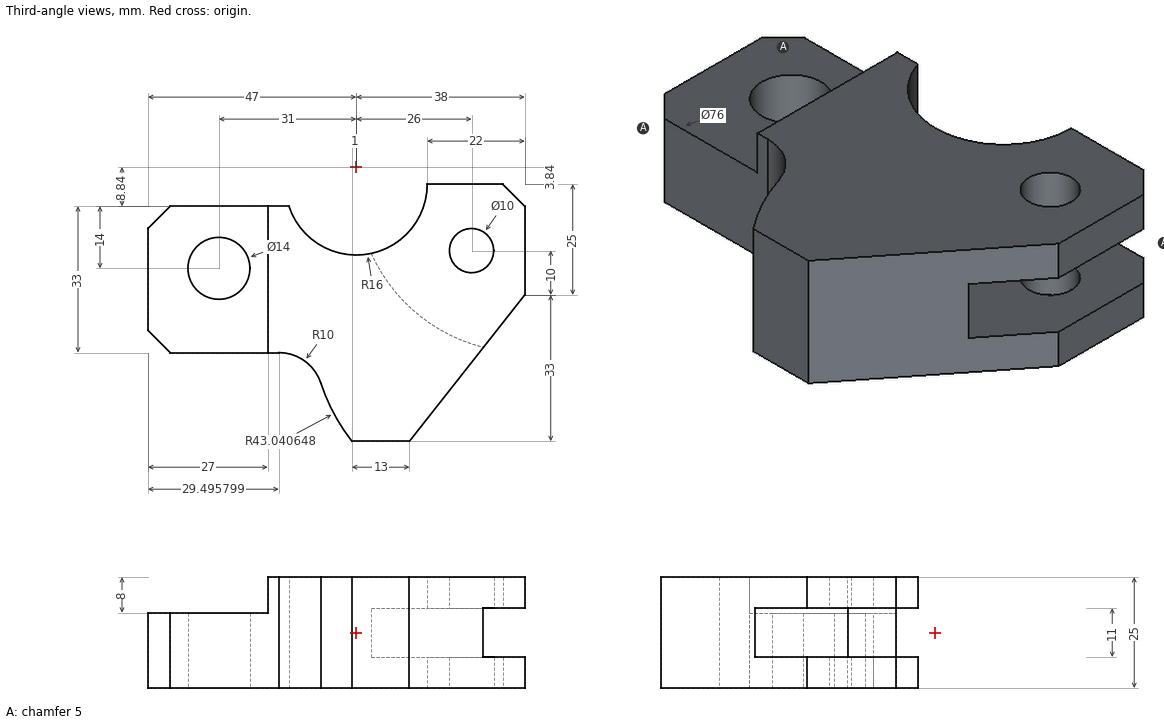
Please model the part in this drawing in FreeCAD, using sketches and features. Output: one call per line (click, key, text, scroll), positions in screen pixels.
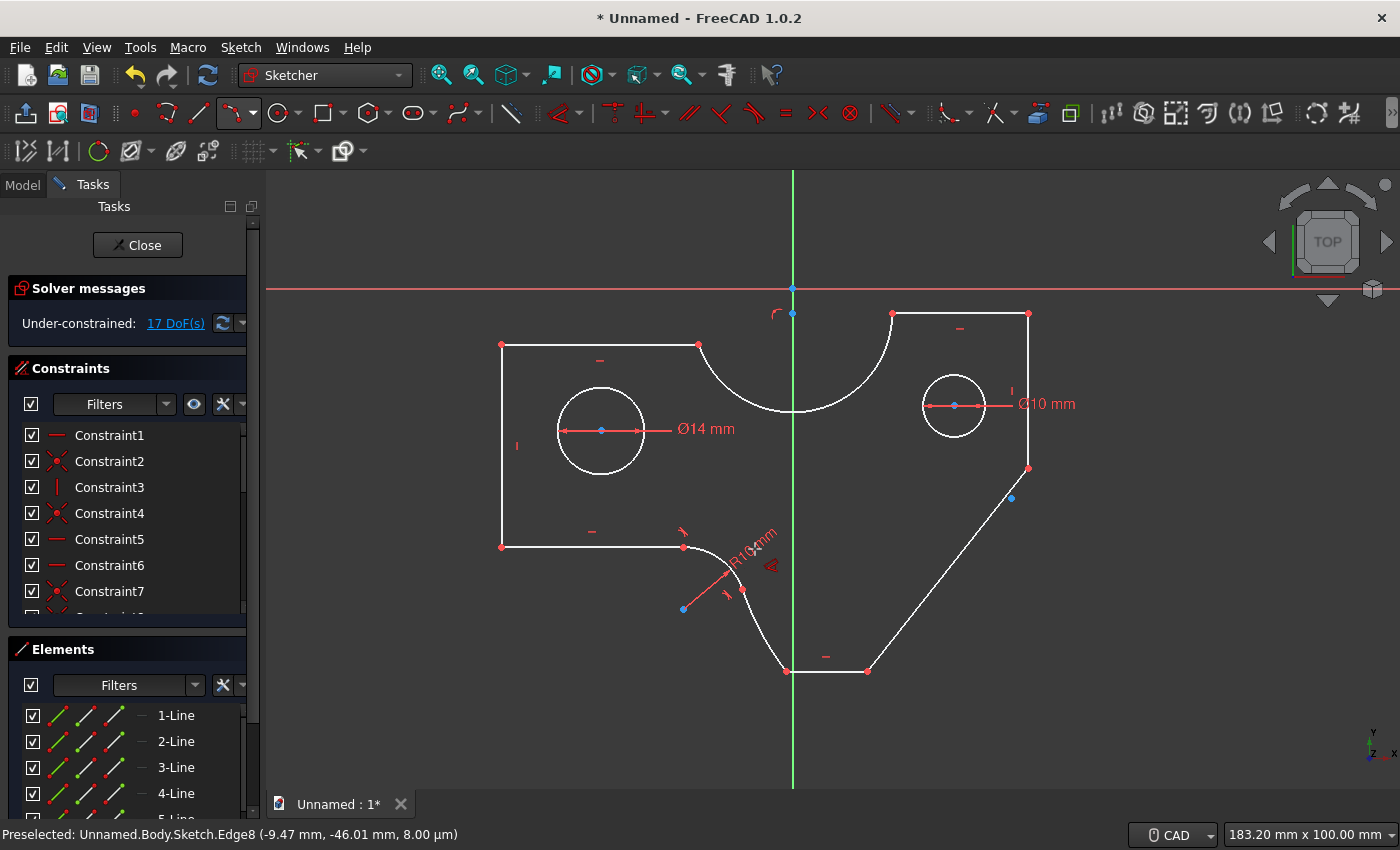
click(753, 616)
click(724, 629)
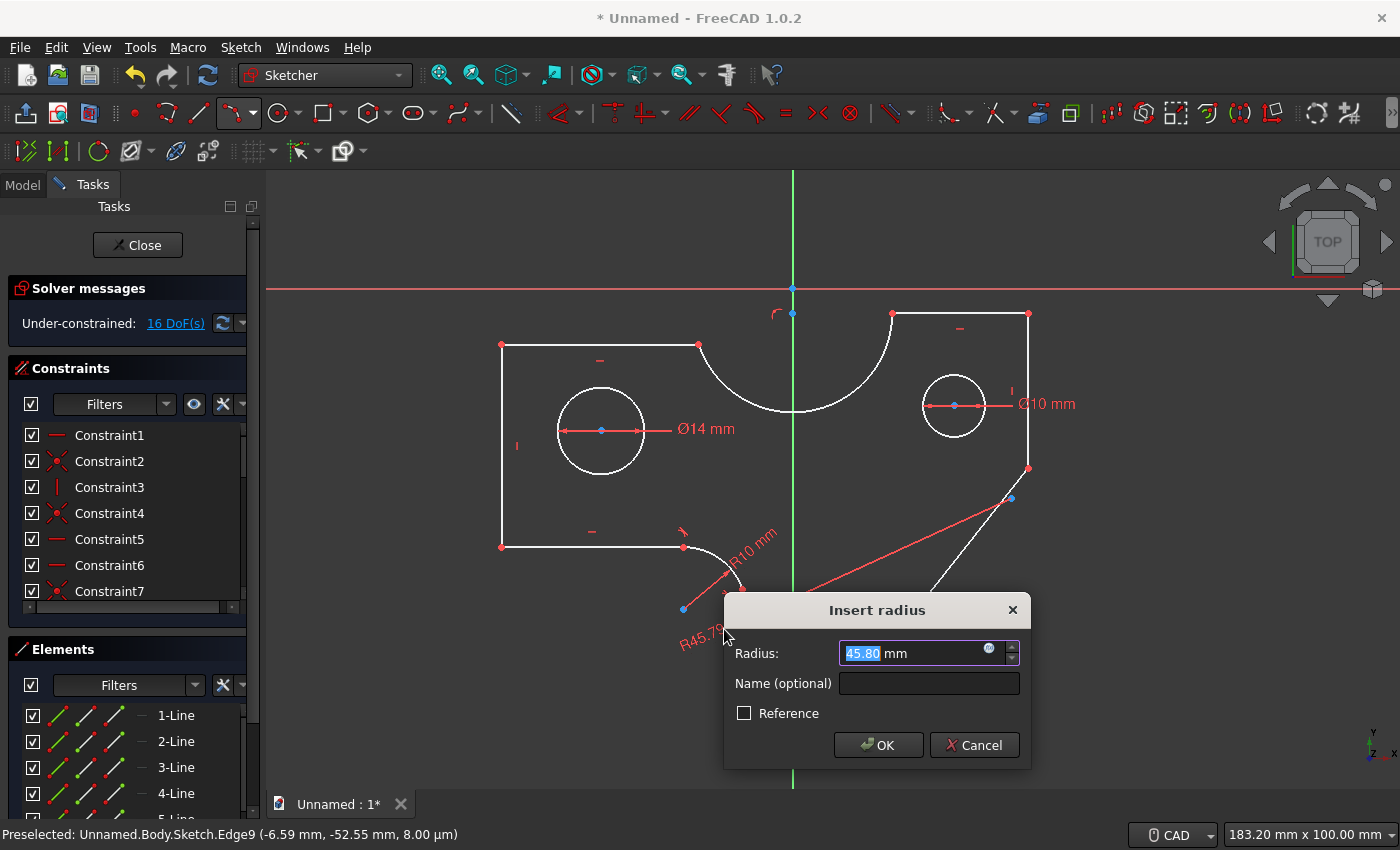
text(43.040648)
key(Return)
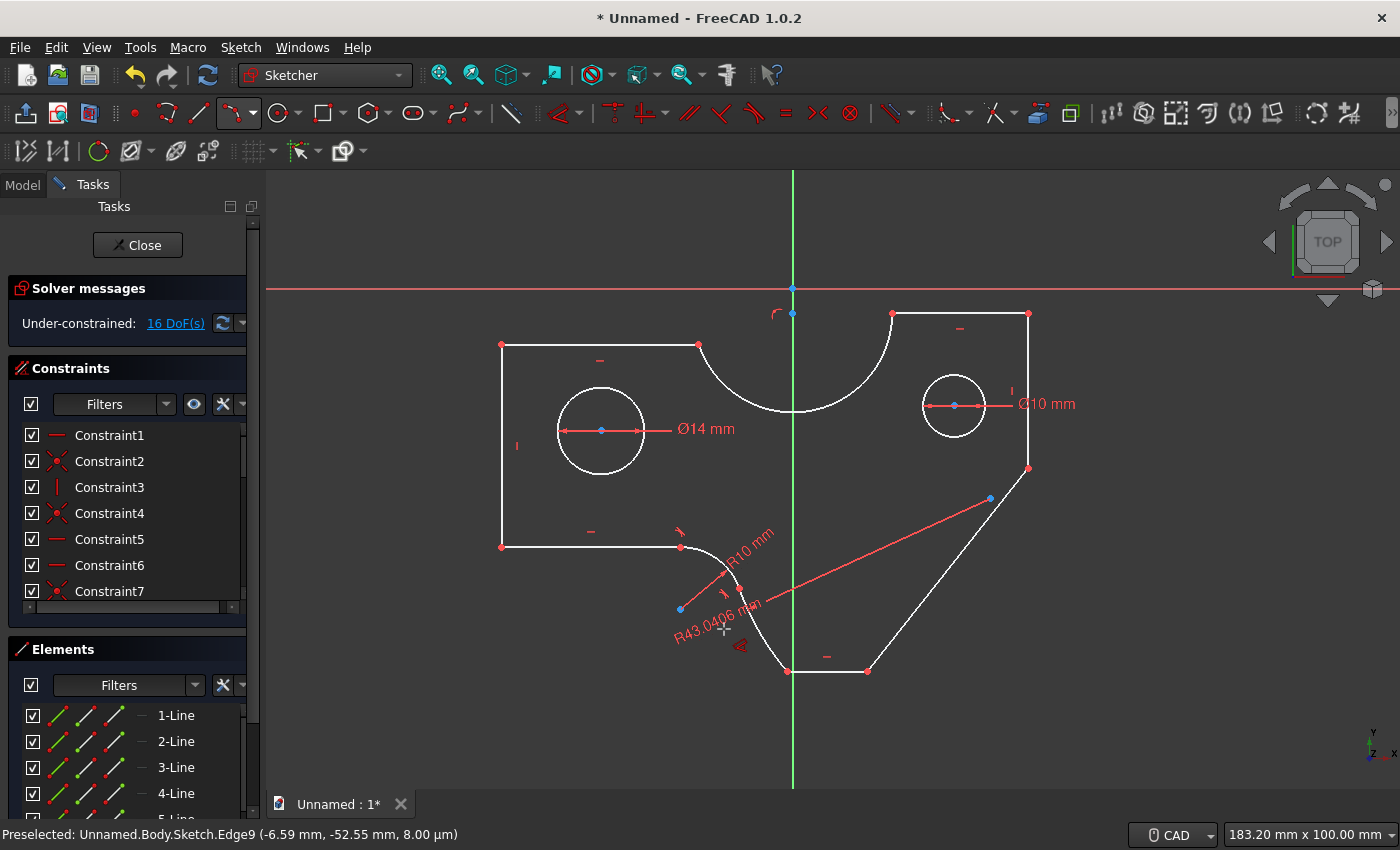
click(754, 404)
click(741, 433)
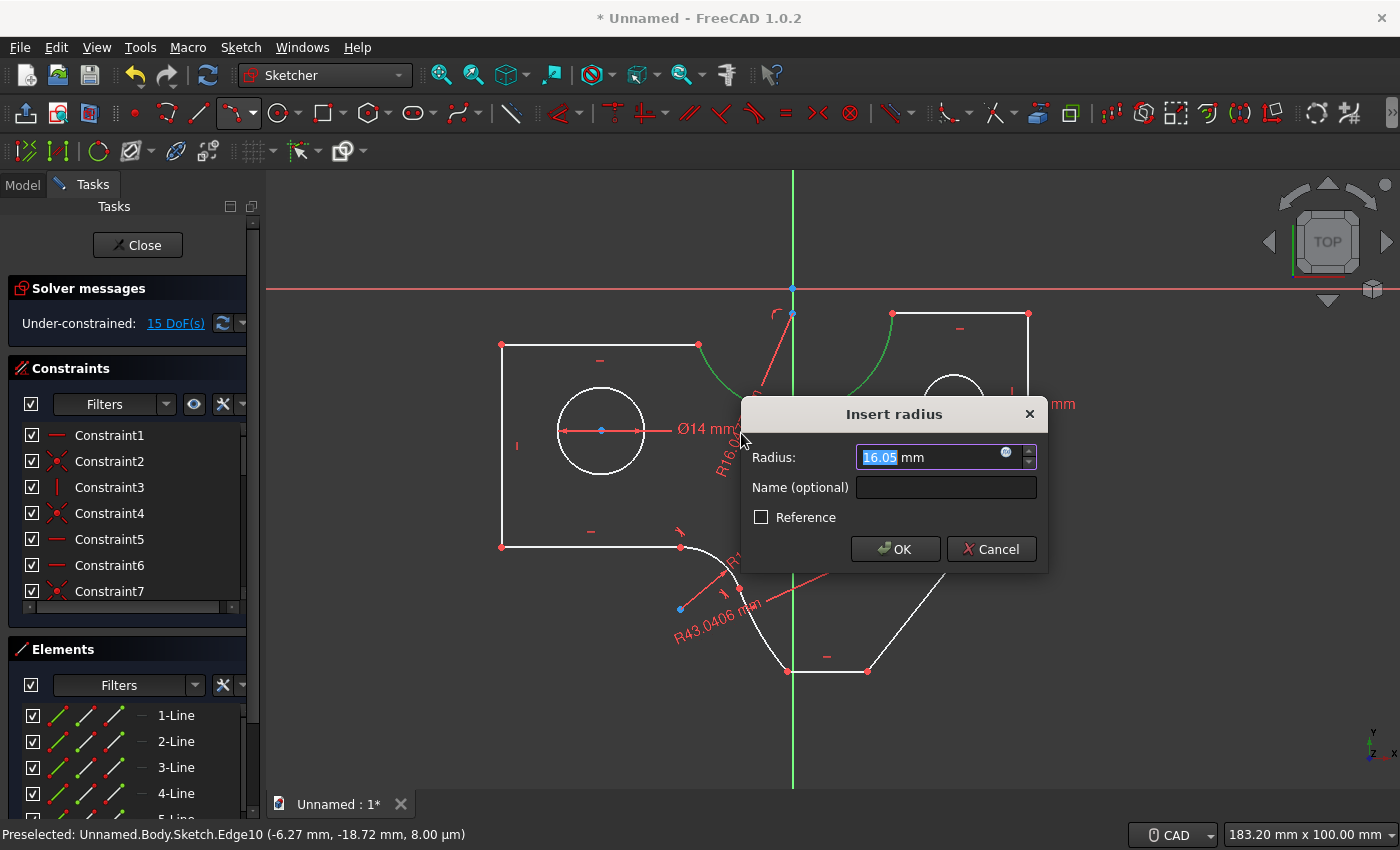
text(16)
key(Return)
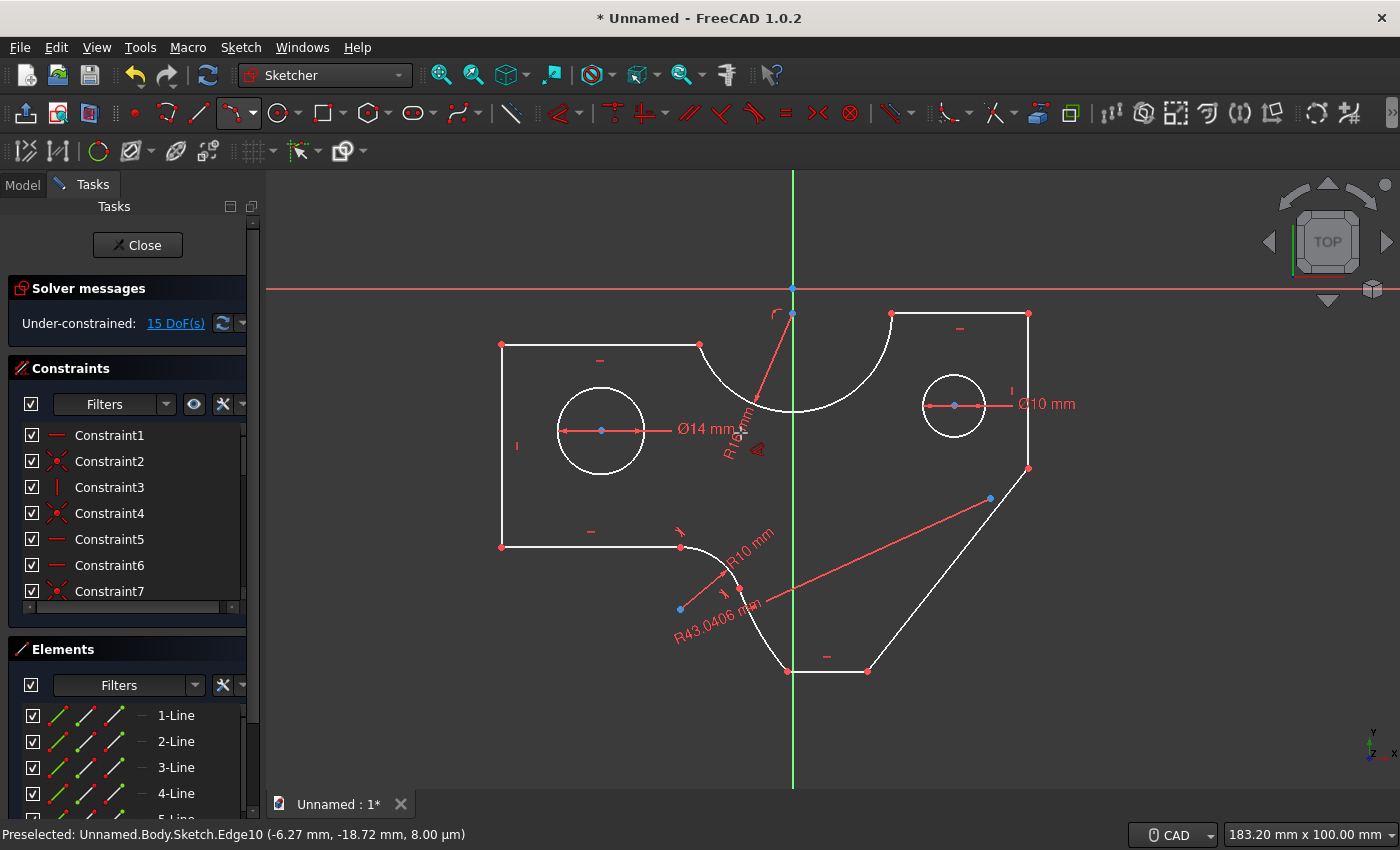
click(502, 405)
click(468, 446)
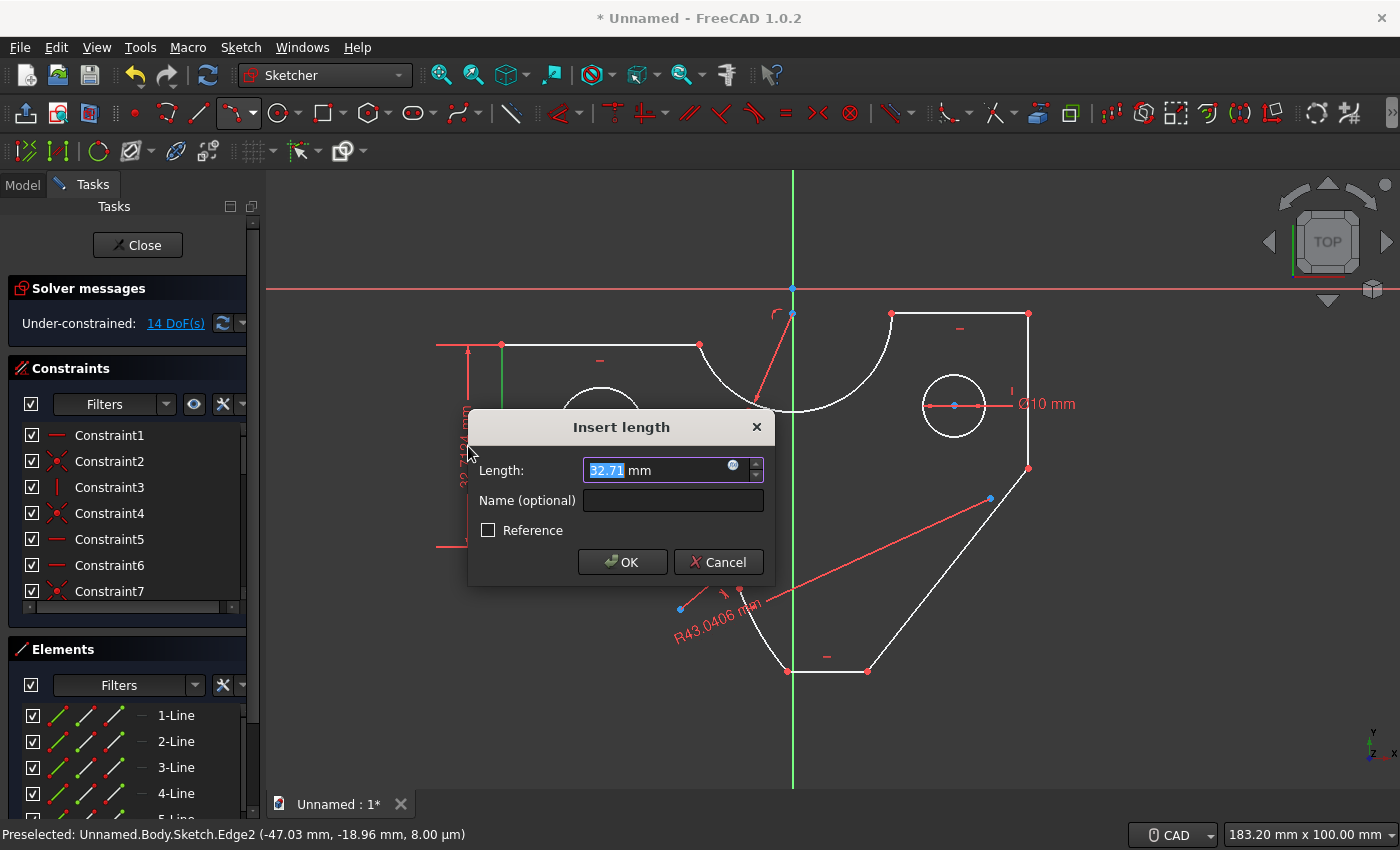
text(33)
key(Return)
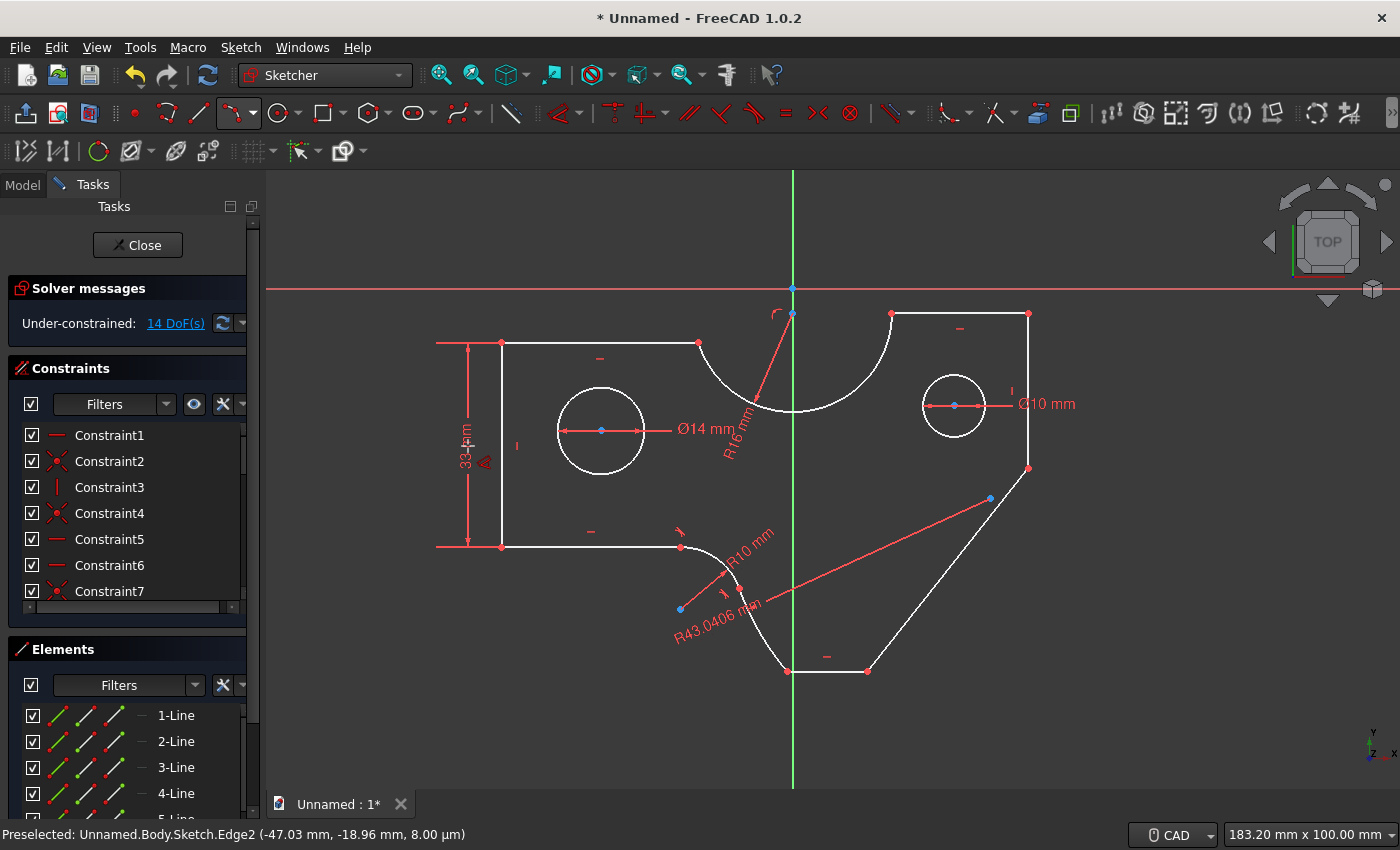
click(811, 672)
click(827, 706)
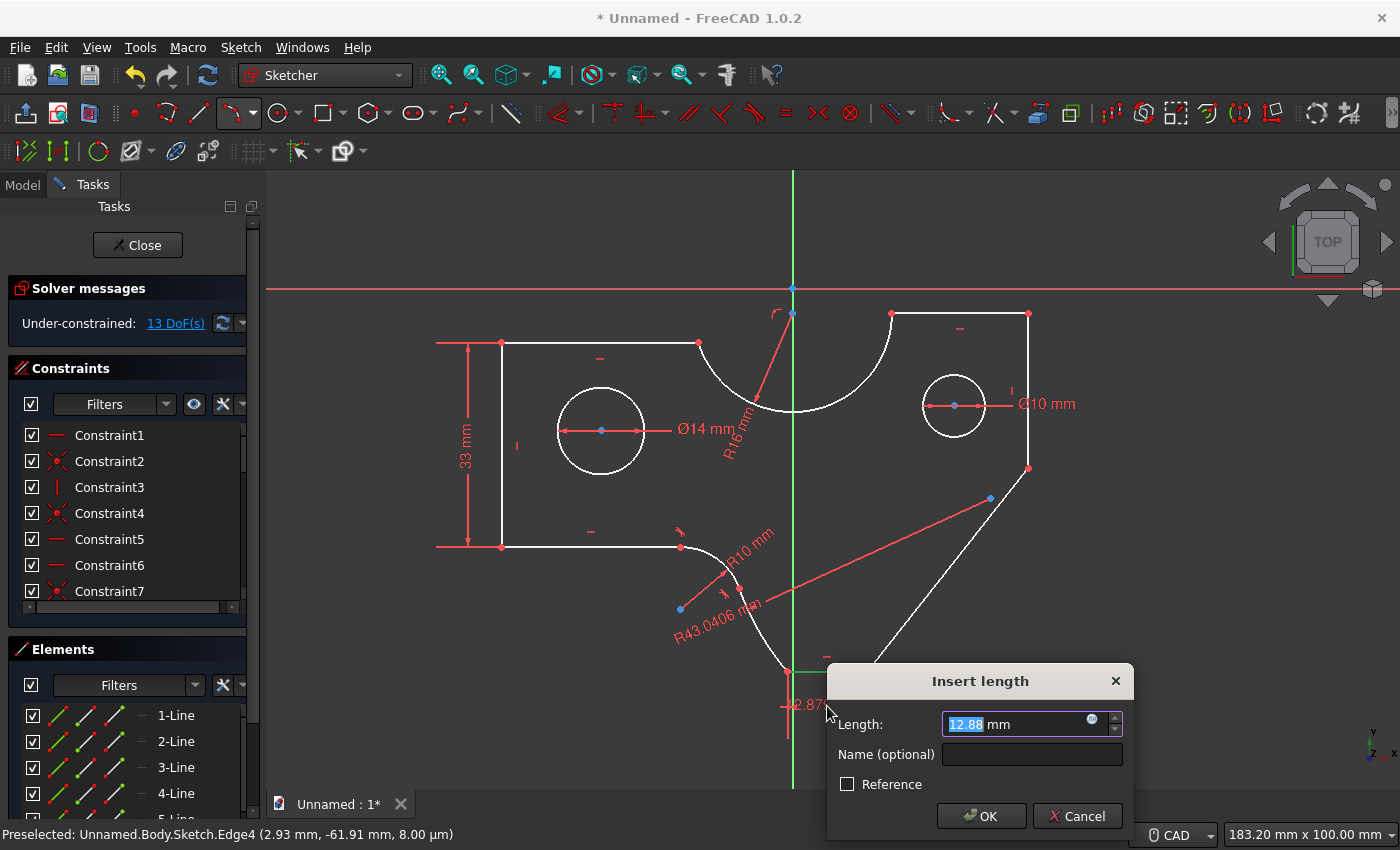
text(13)
key(Return)